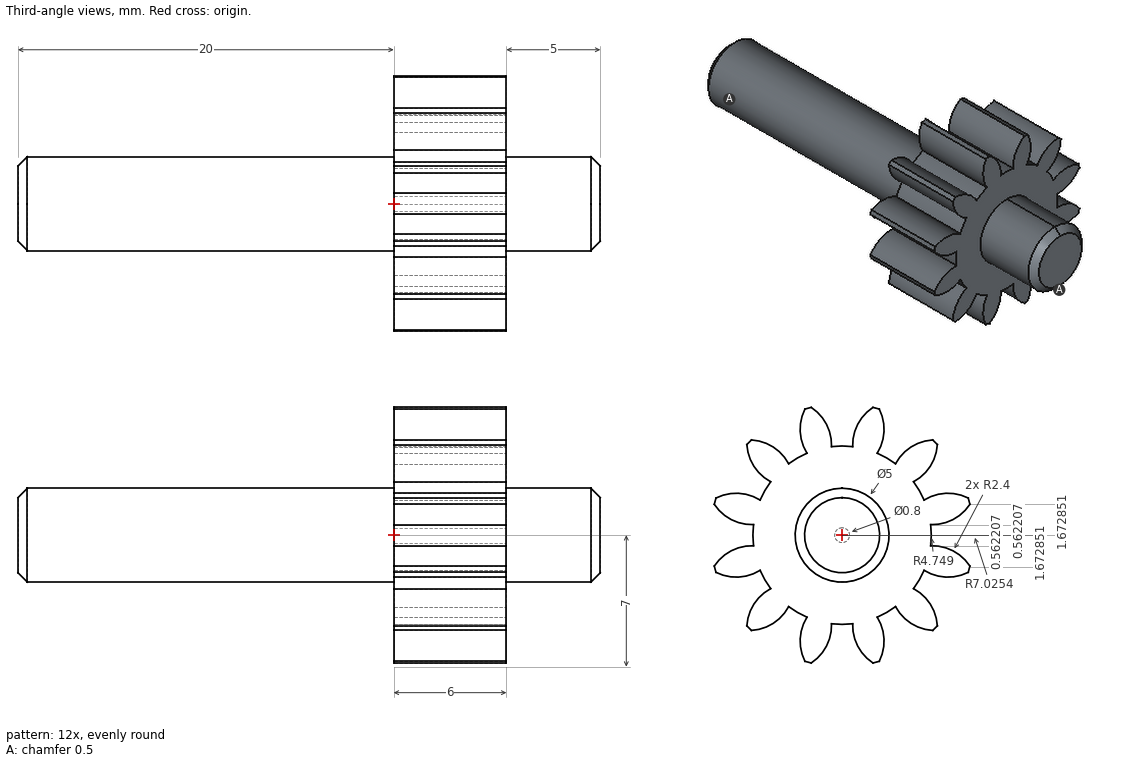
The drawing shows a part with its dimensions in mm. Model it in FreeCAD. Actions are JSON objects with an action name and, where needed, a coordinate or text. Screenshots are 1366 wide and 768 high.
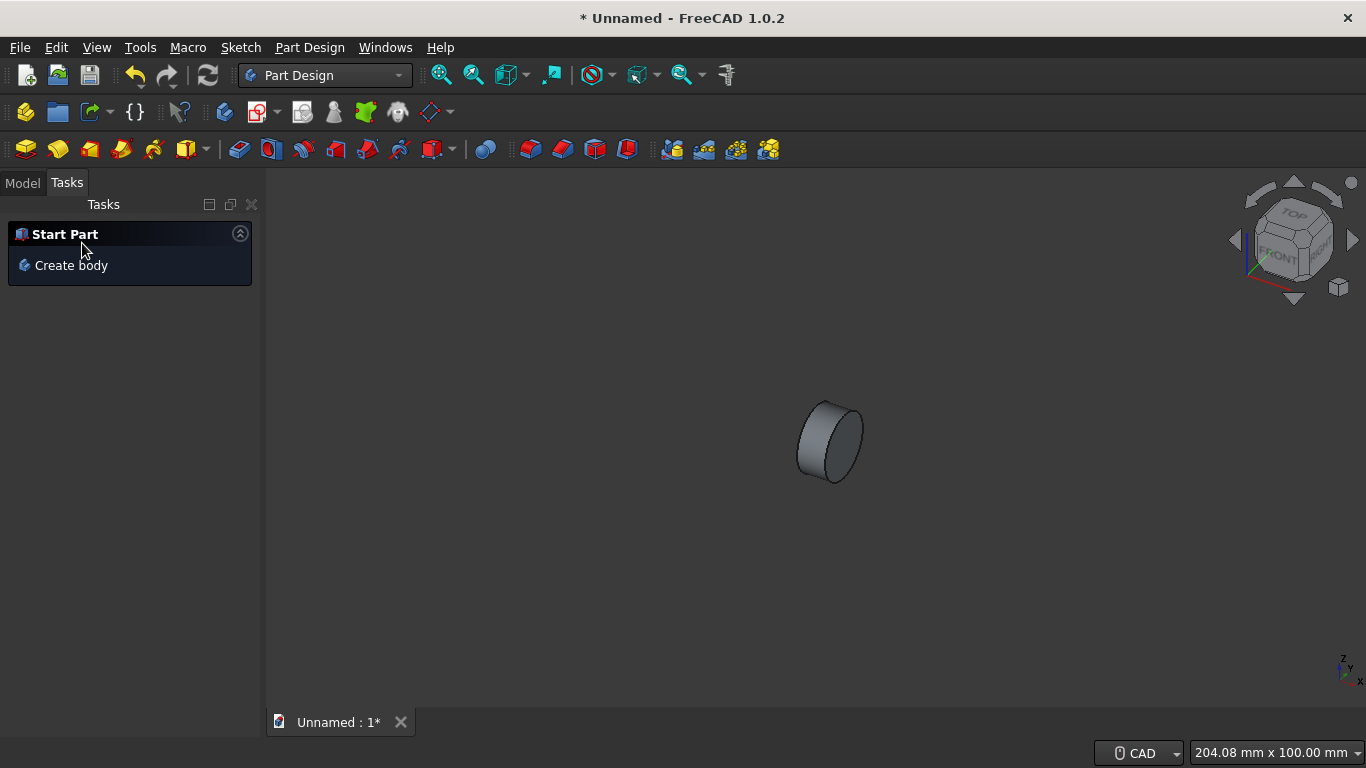
{"action": "key", "text": "v f"}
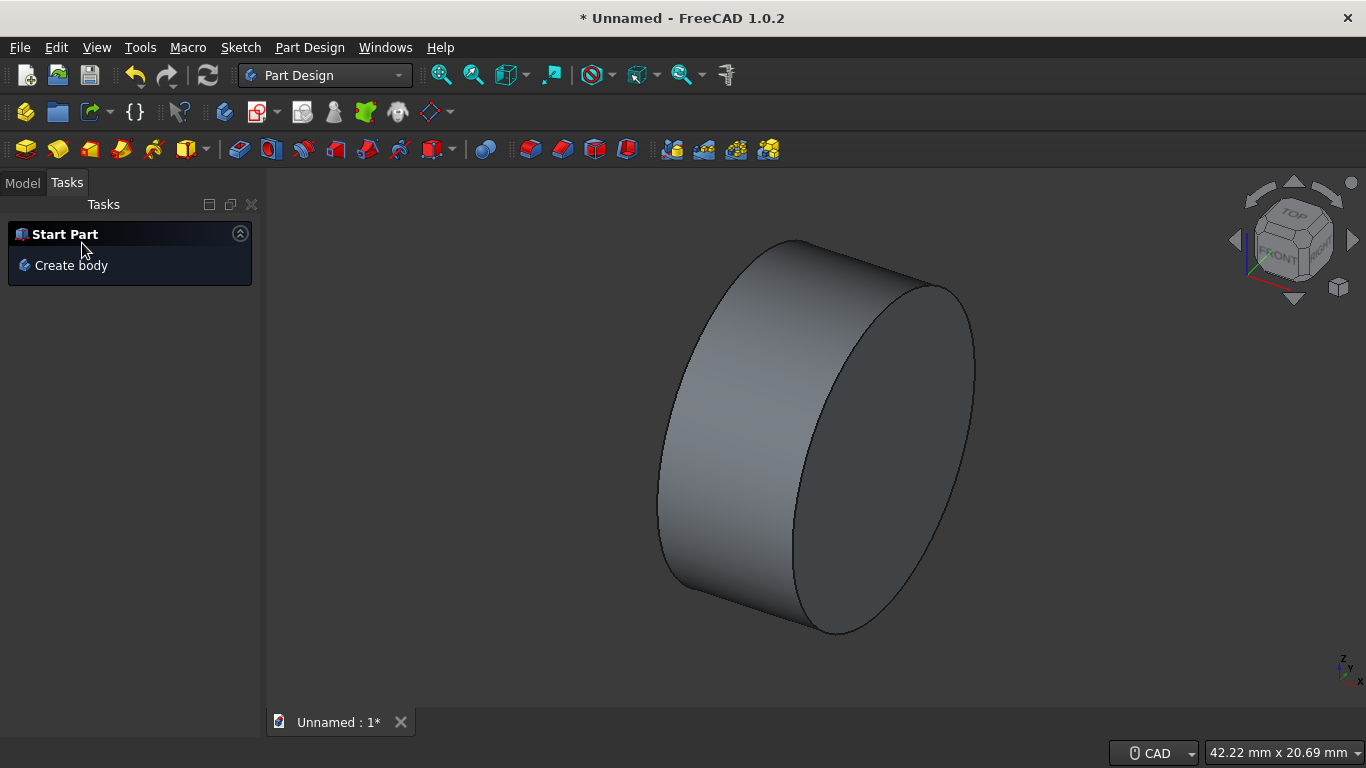
{"action": "left_click", "coordinate": [258, 112]}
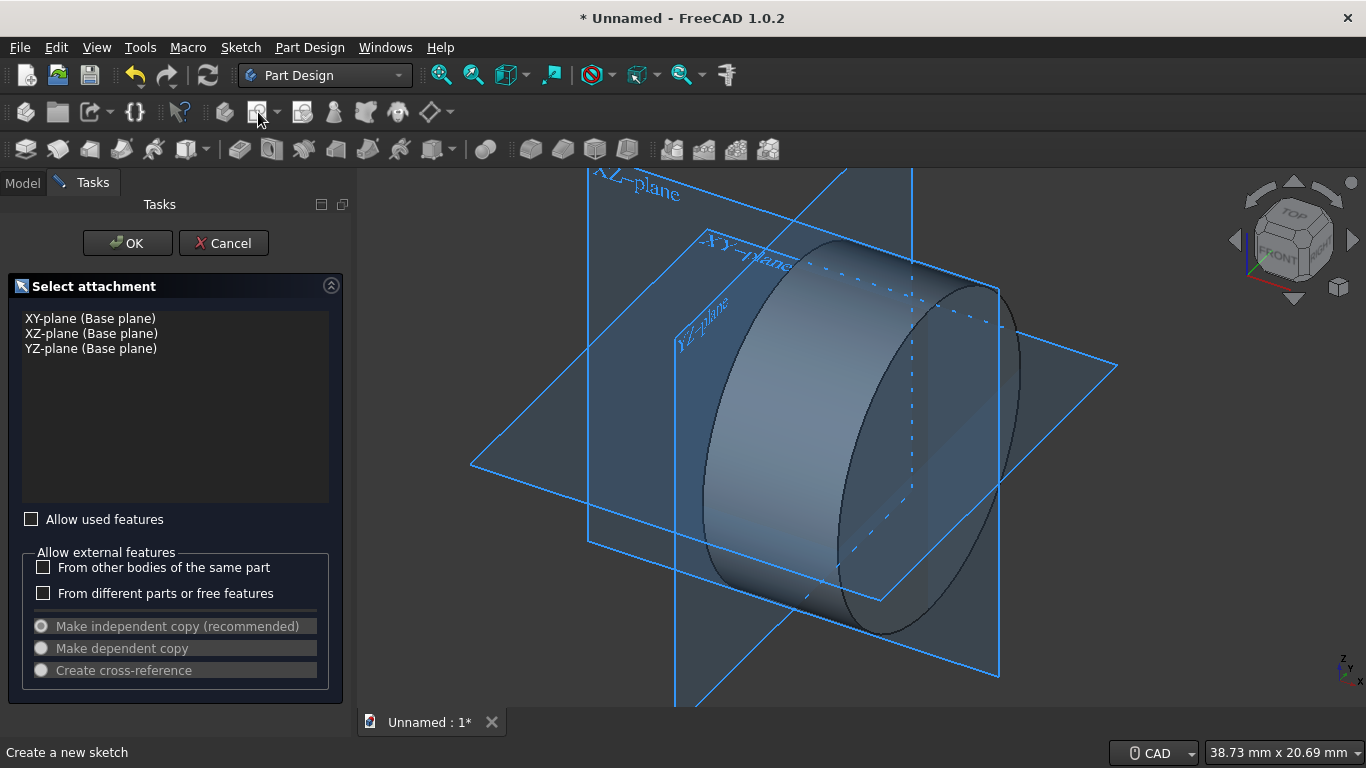
{"action": "left_click", "coordinate": [82, 348]}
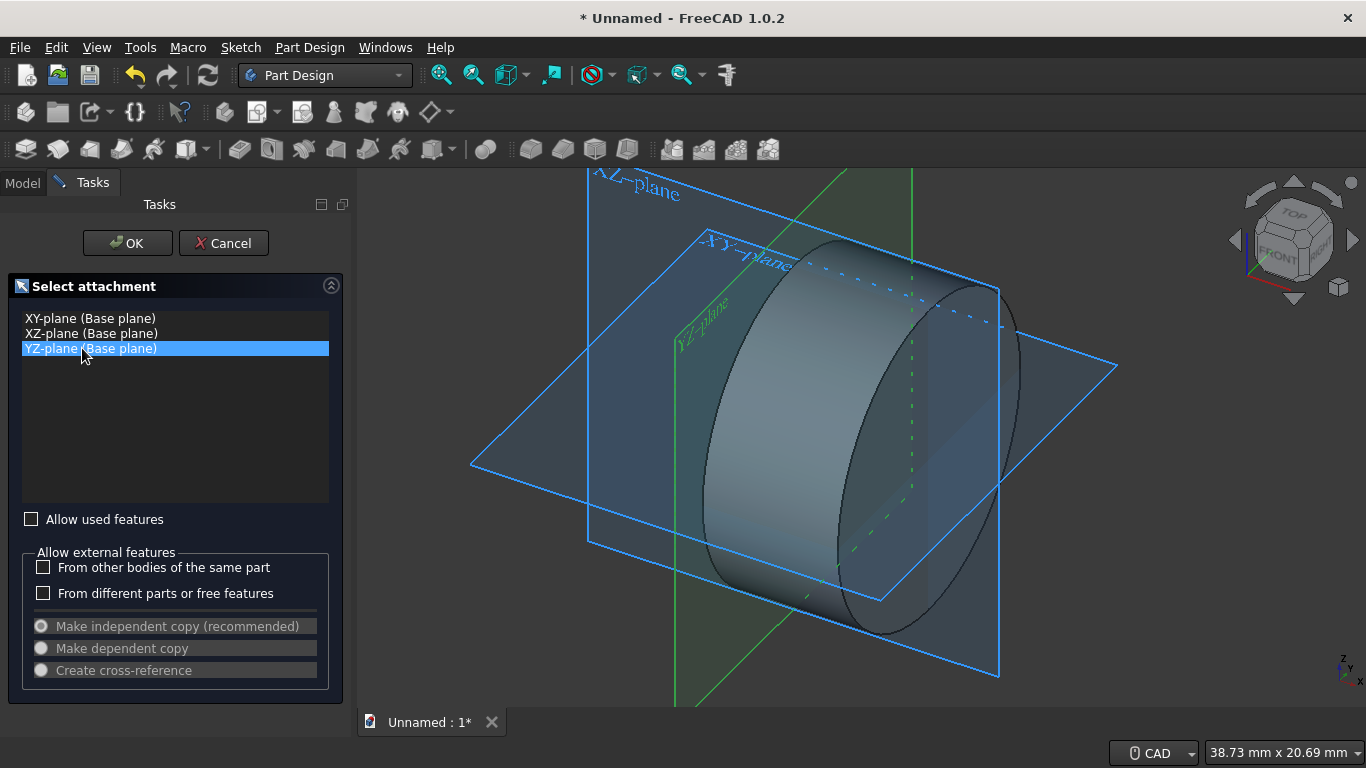
{"action": "left_click", "coordinate": [128, 243]}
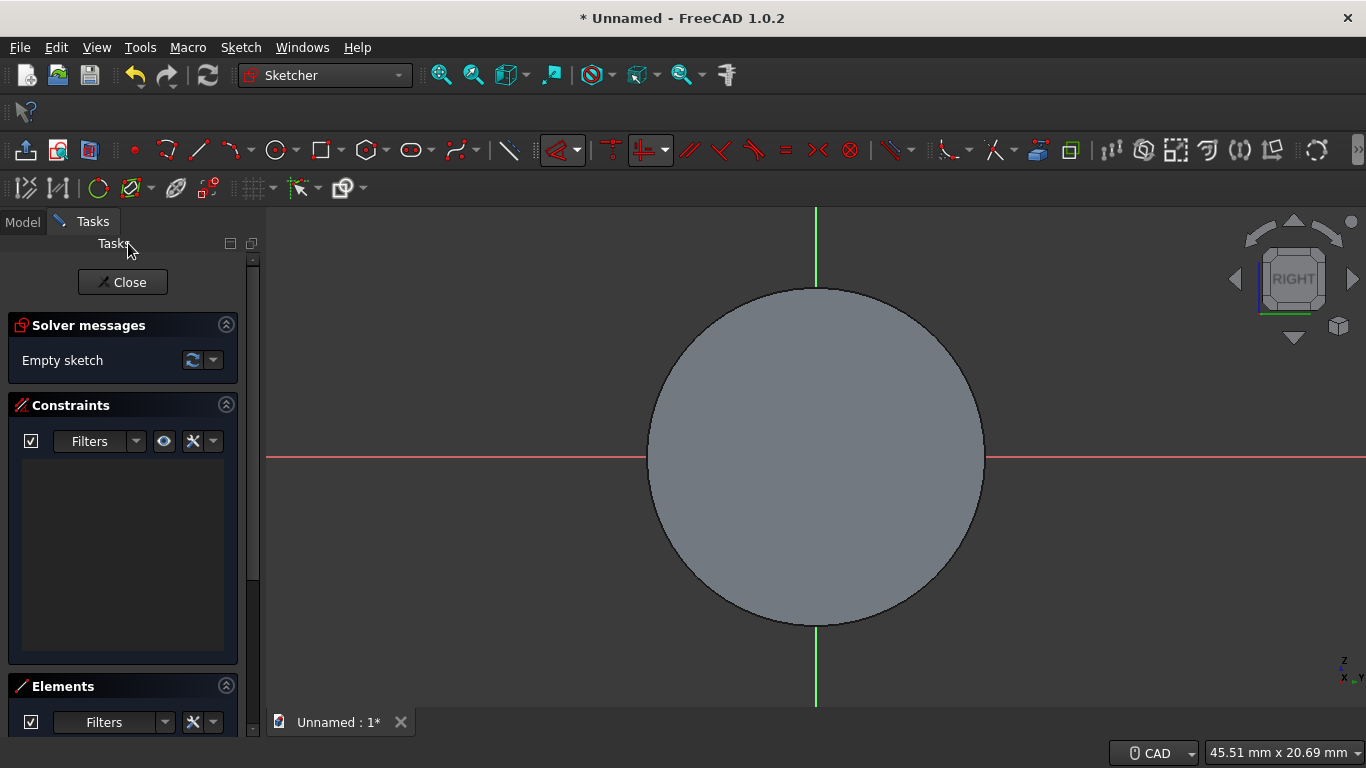
{"action": "left_click", "coordinate": [90, 150]}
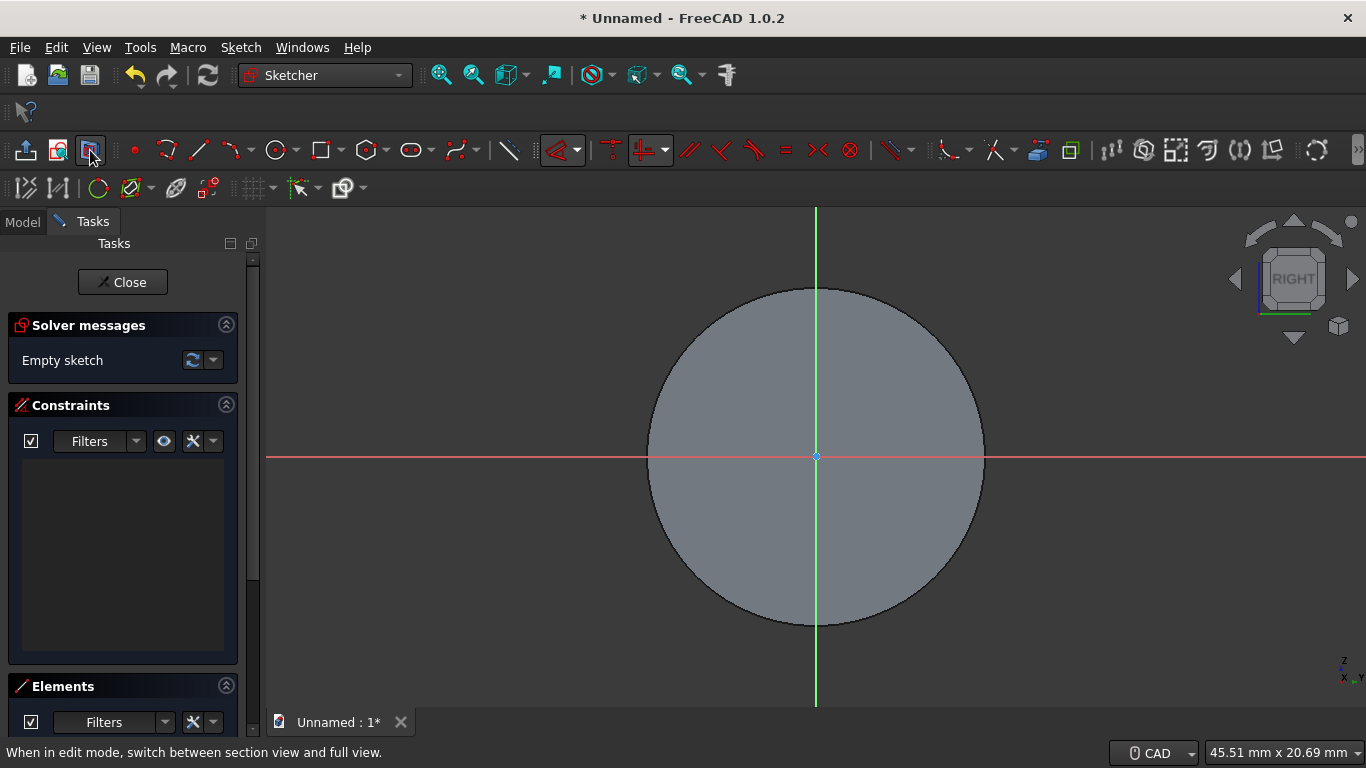
{"action": "scroll", "coordinate": [951, 457], "scroll_direction": "up", "scroll_amount": 7}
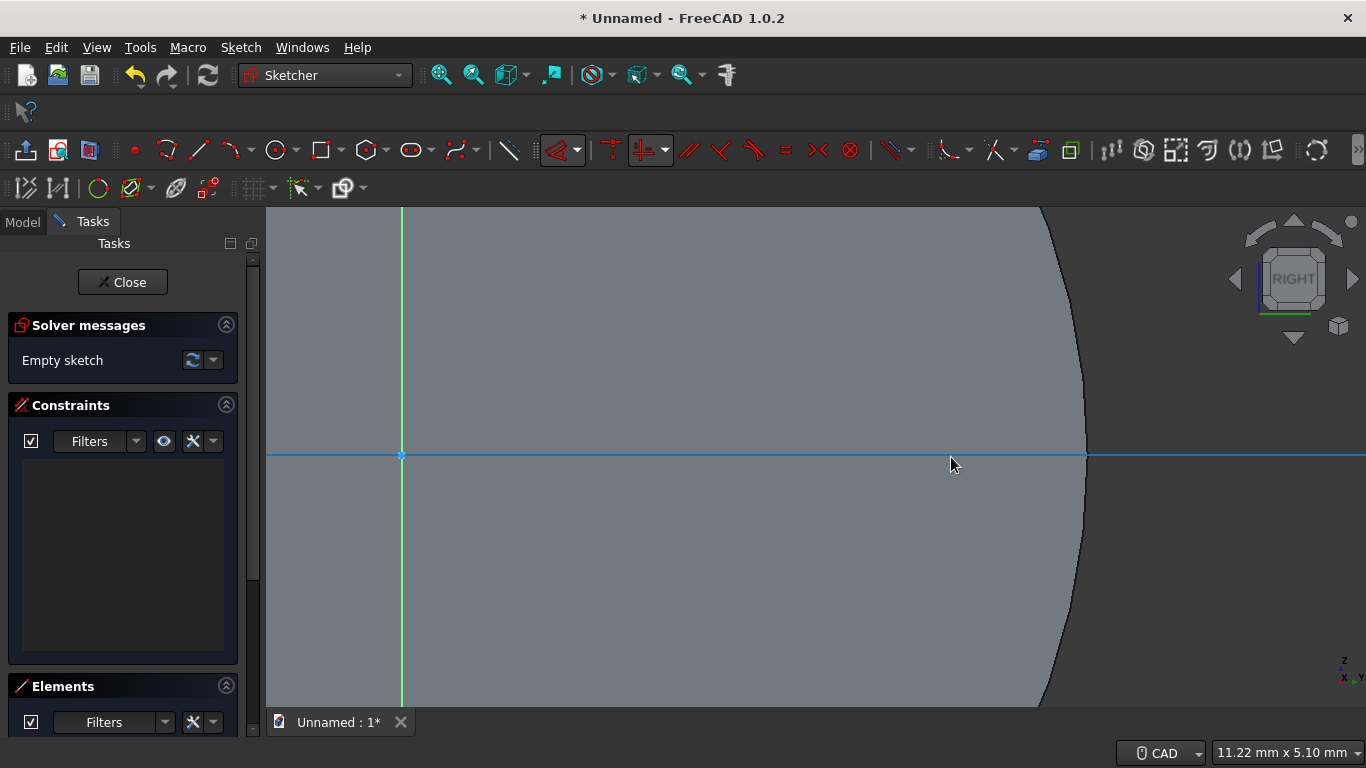
{"action": "left_click", "coordinate": [232, 150]}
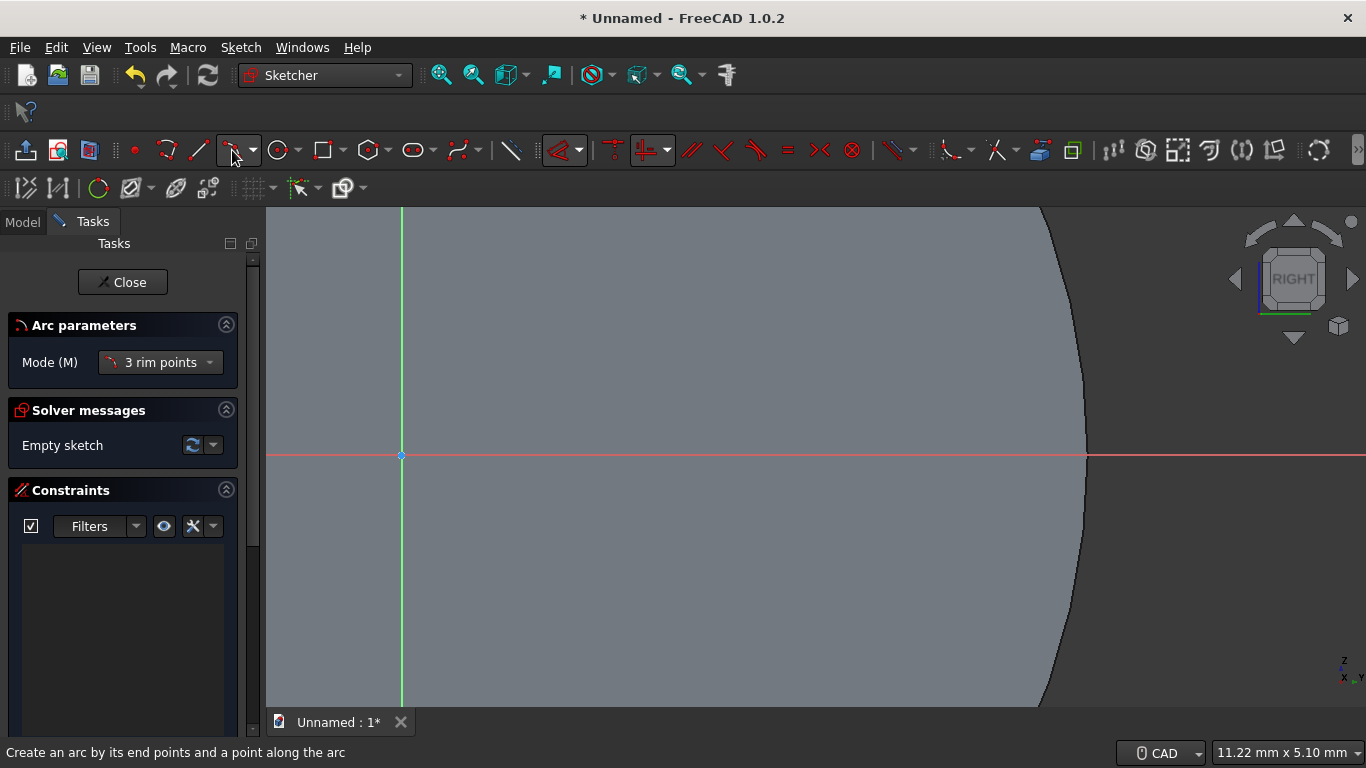
{"action": "left_click", "coordinate": [864, 400]}
{"action": "left_click", "coordinate": [864, 511]}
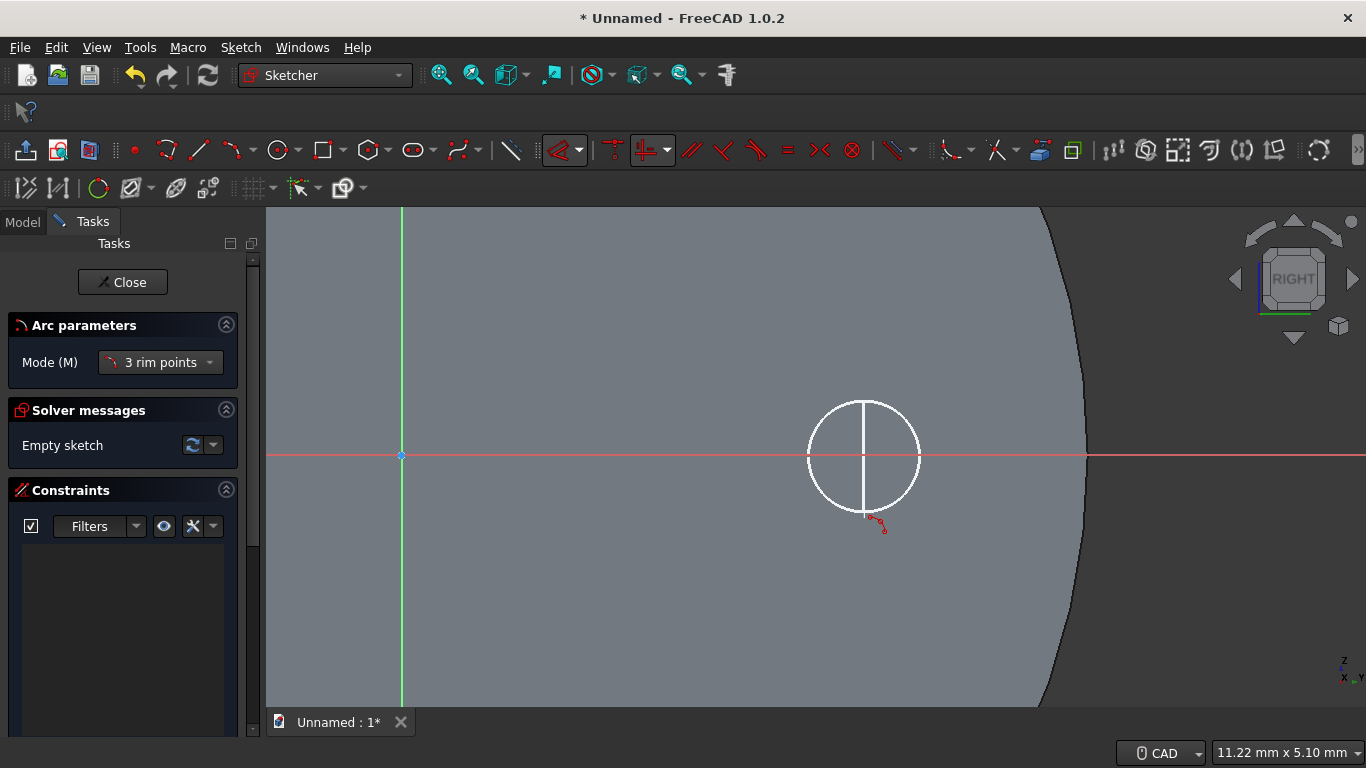
{"action": "scroll", "coordinate": [867, 467], "scroll_direction": "up", "scroll_amount": 9}